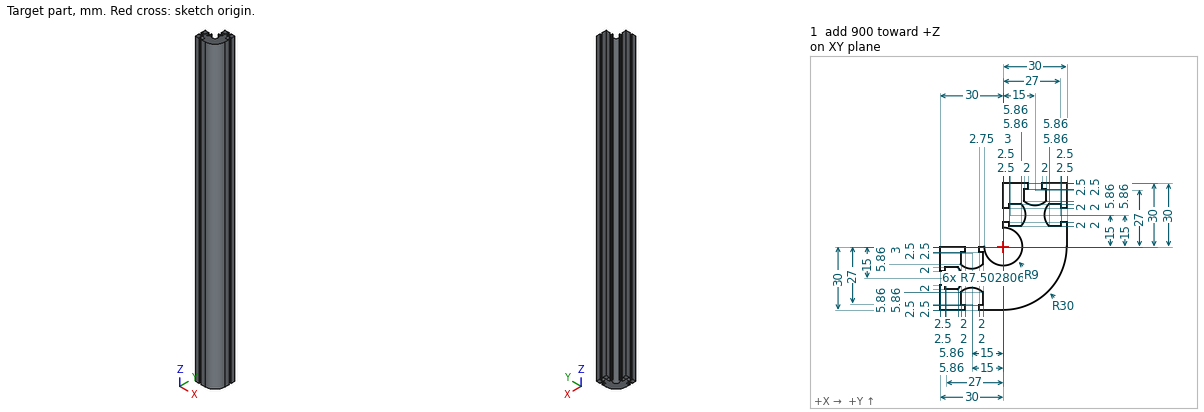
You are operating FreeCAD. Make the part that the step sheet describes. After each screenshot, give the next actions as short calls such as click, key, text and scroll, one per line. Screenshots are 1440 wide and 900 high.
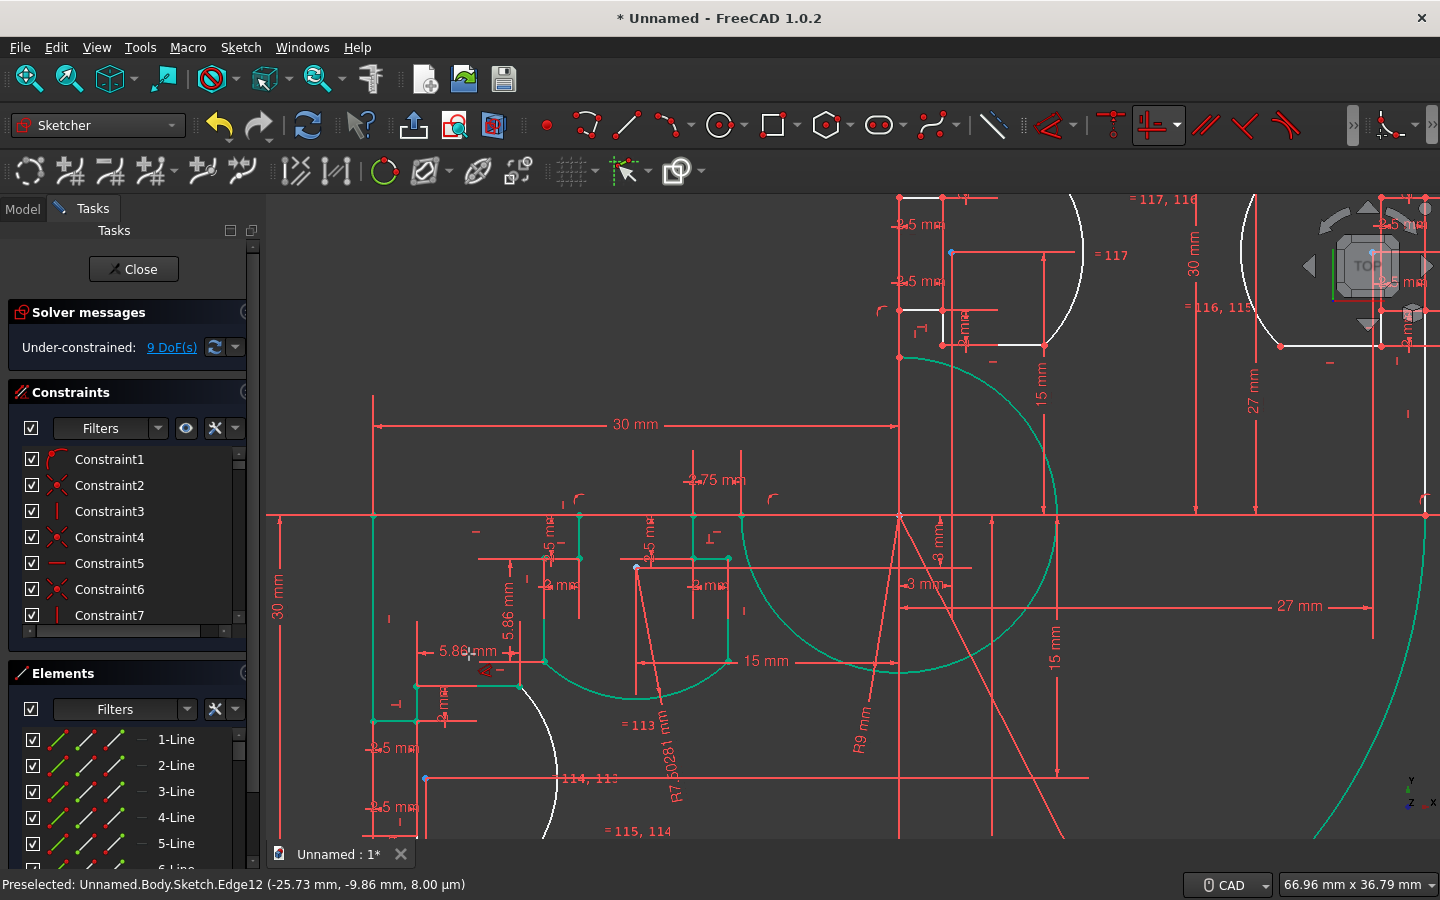
scroll(718, 517, down, 5)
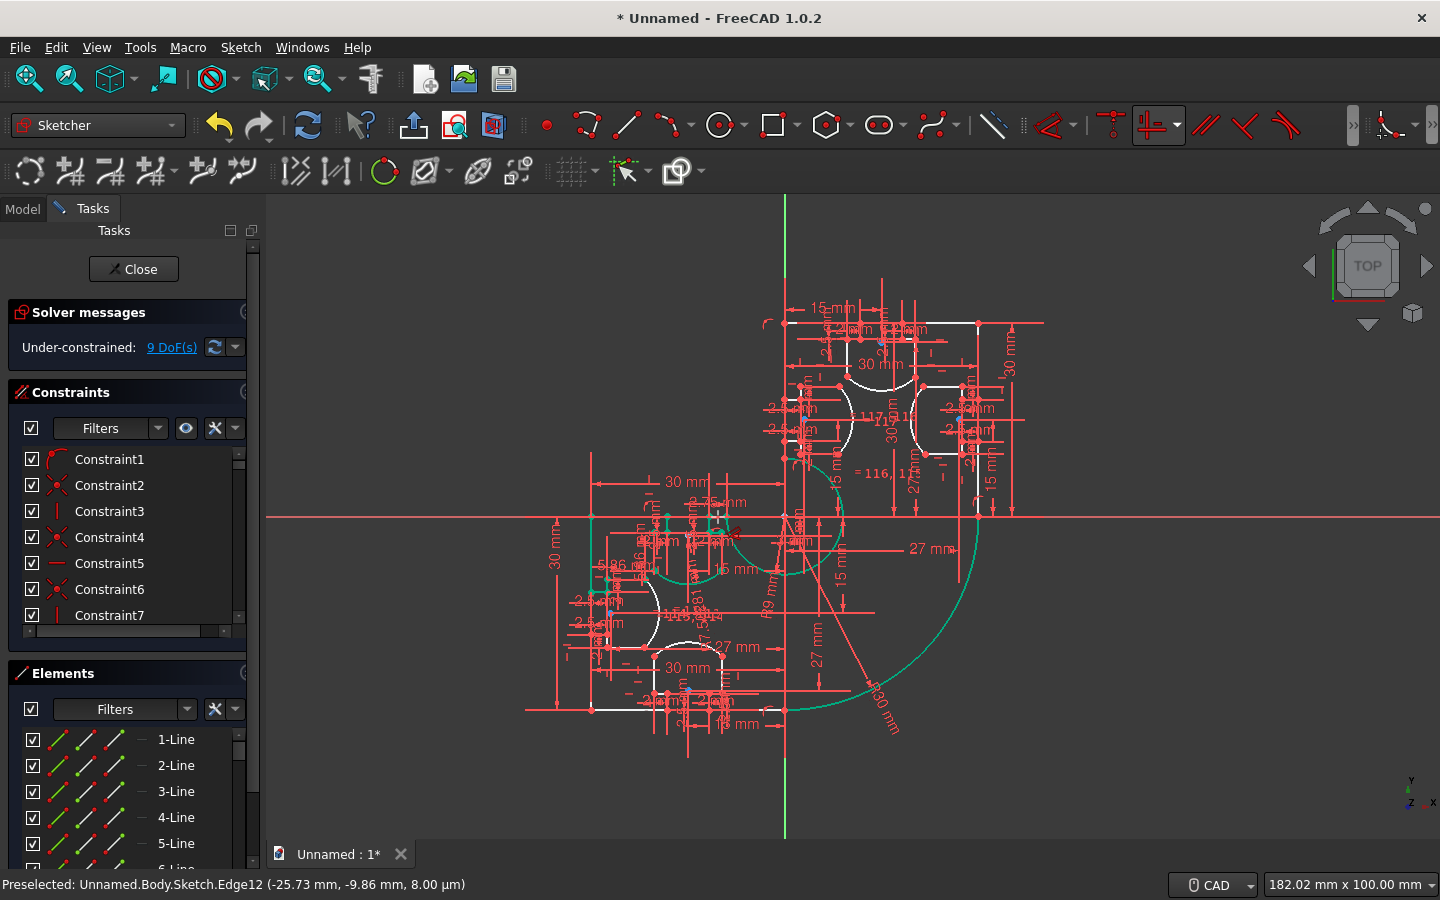
scroll(634, 648, up, 2)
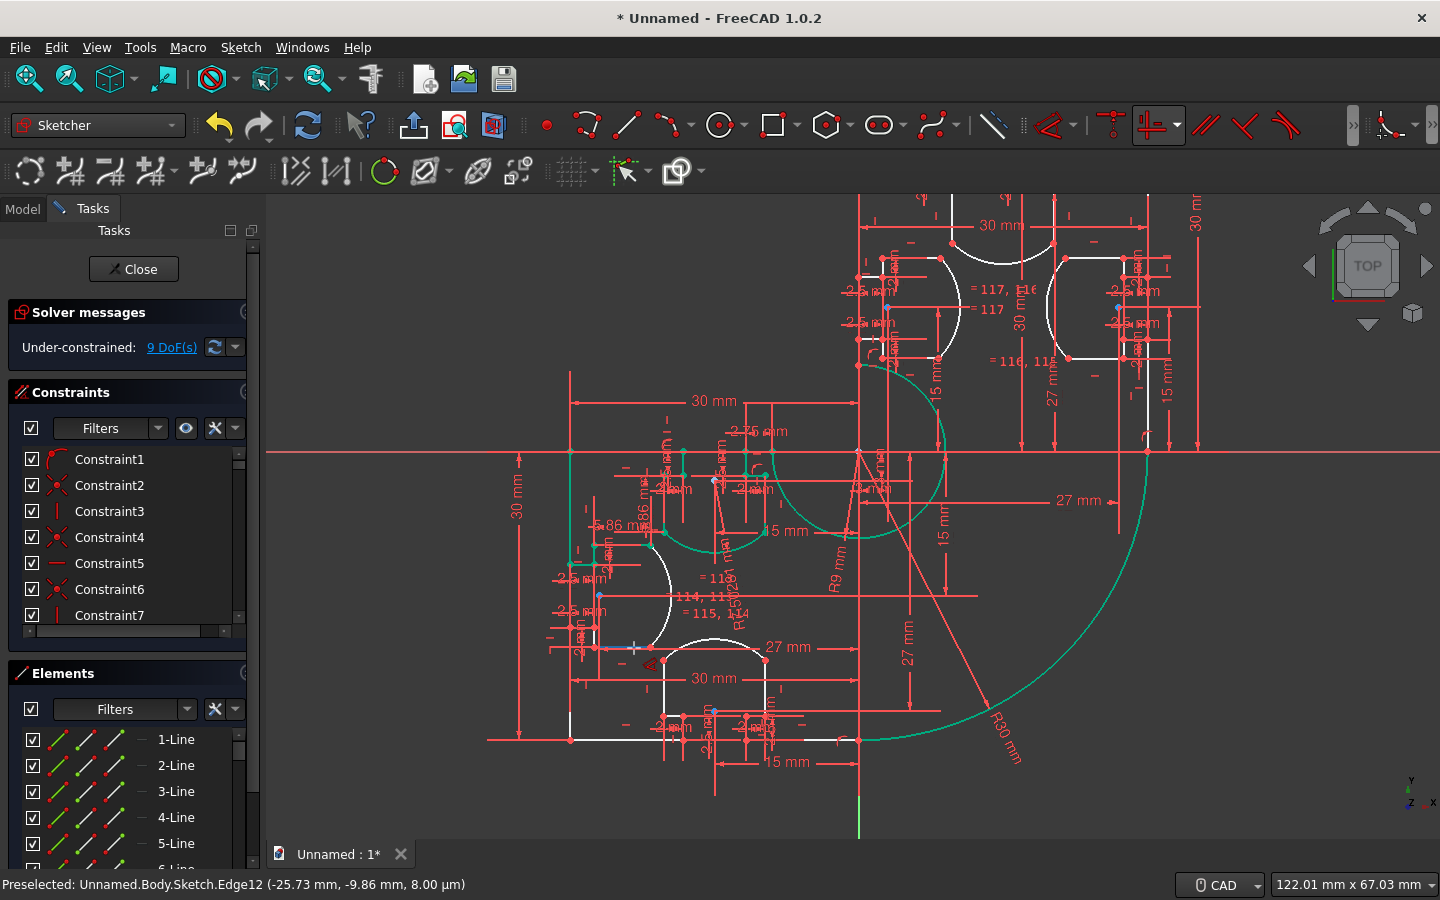
click(633, 647)
click(622, 681)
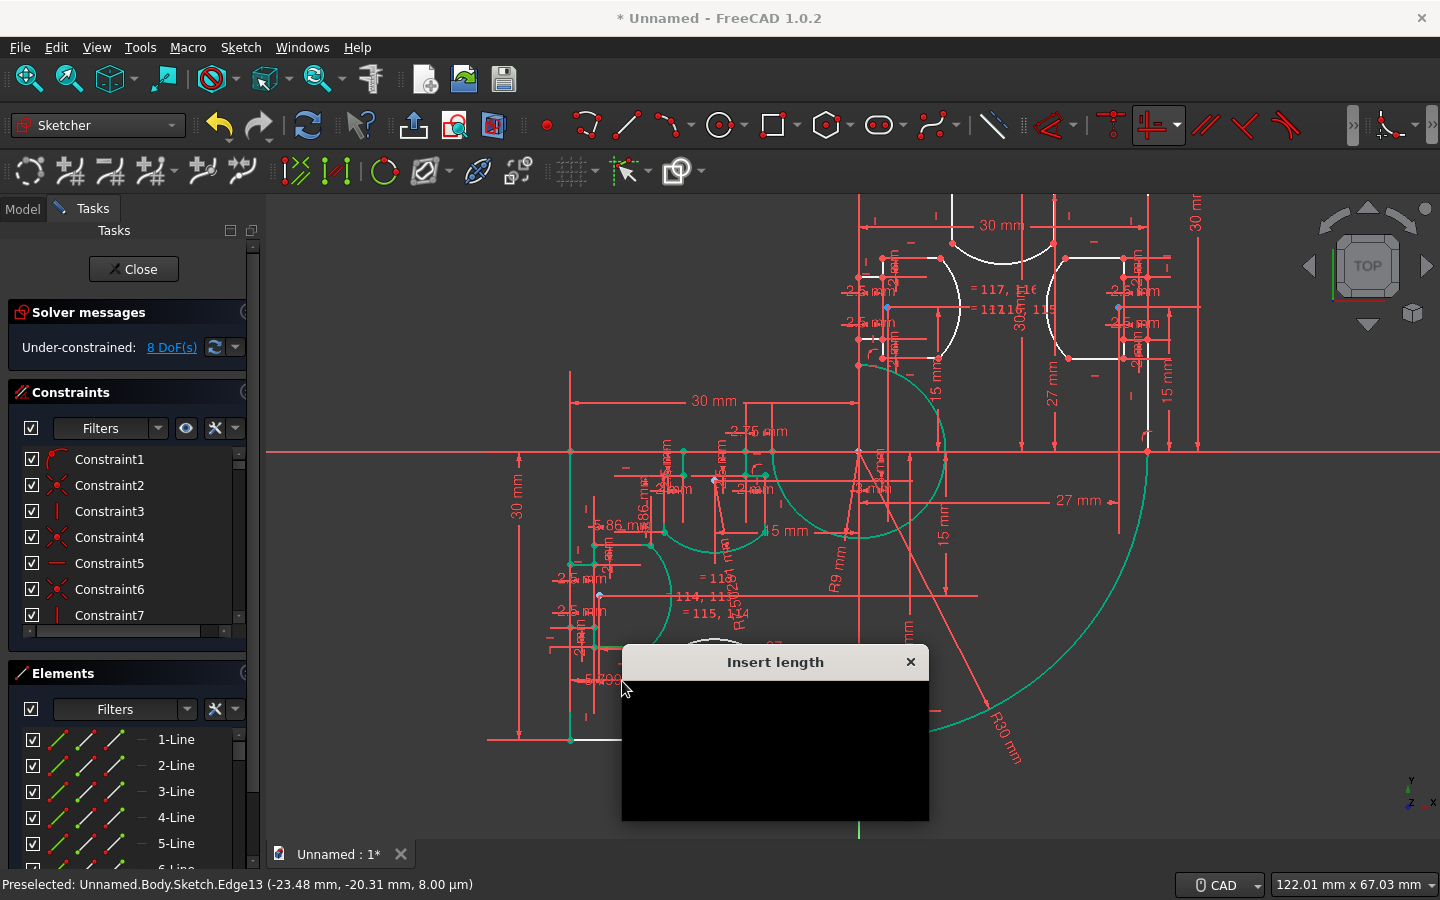
text(5.86)
key(Return)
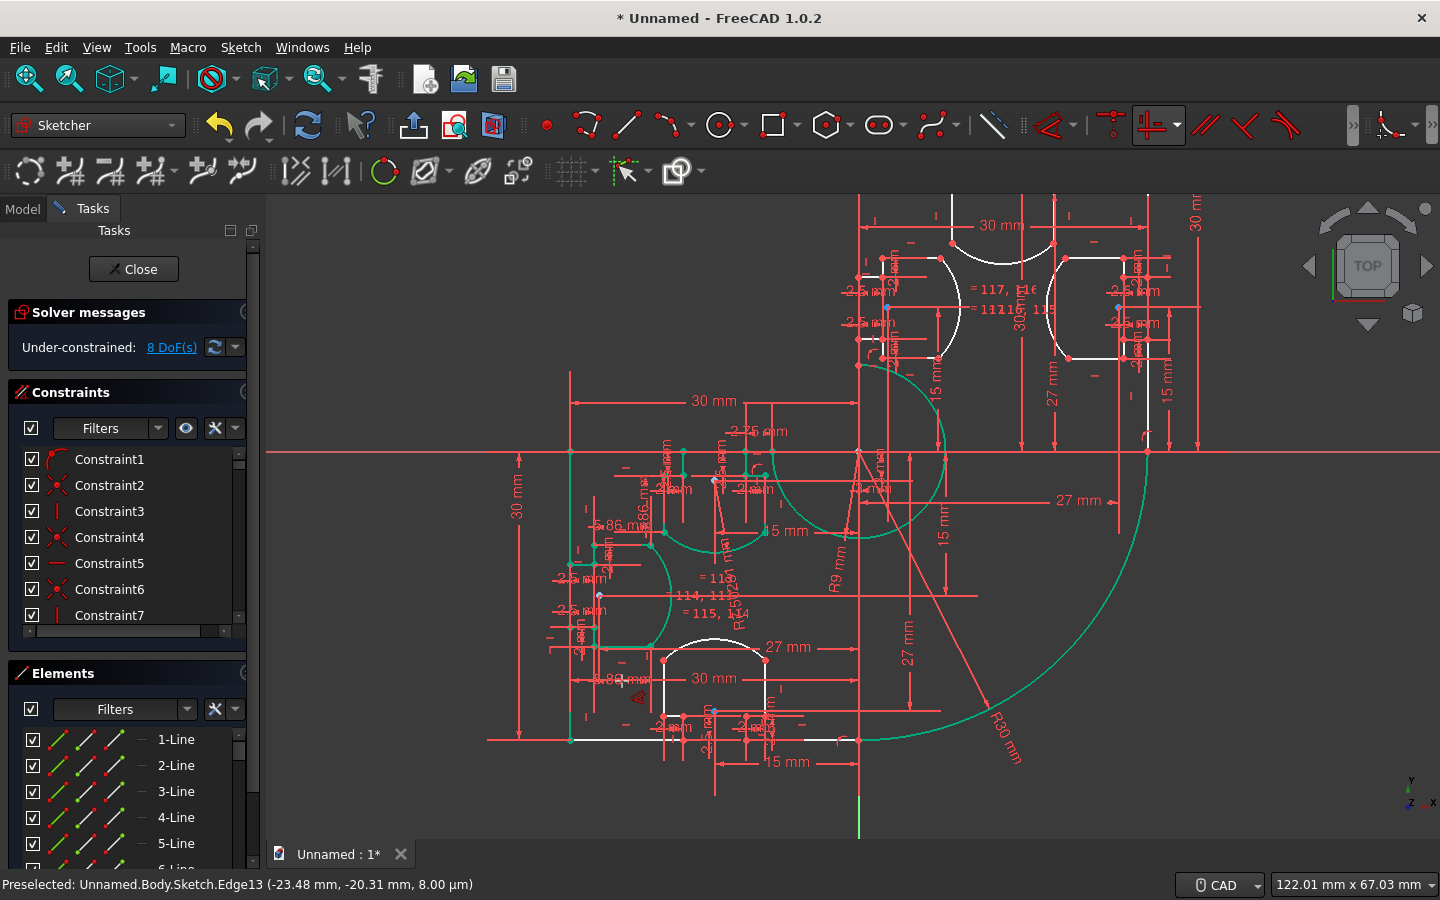
click(664, 699)
click(630, 708)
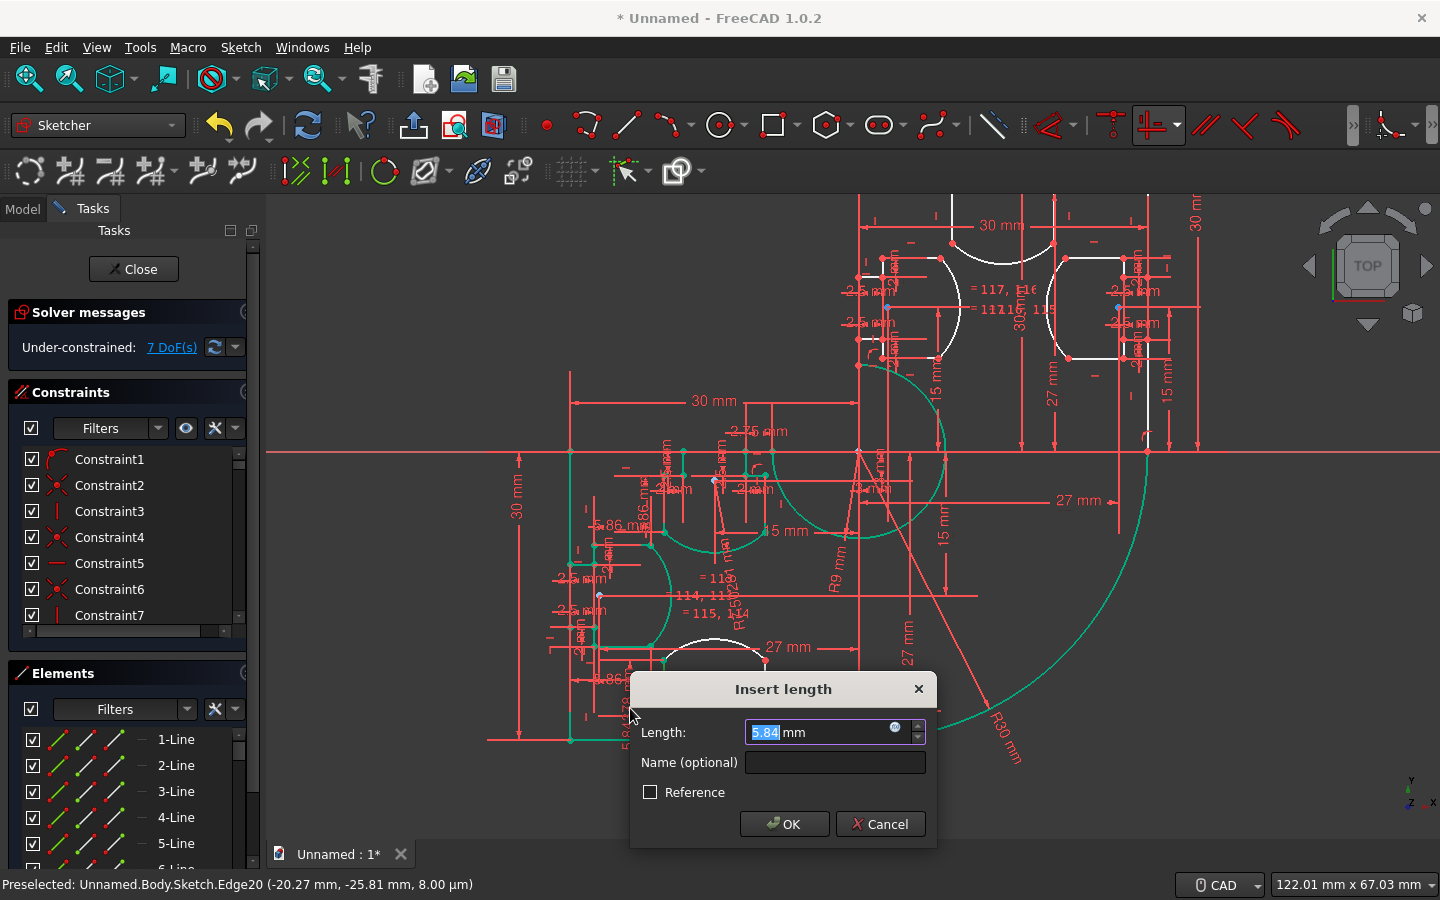
text(5.86)
key(Return)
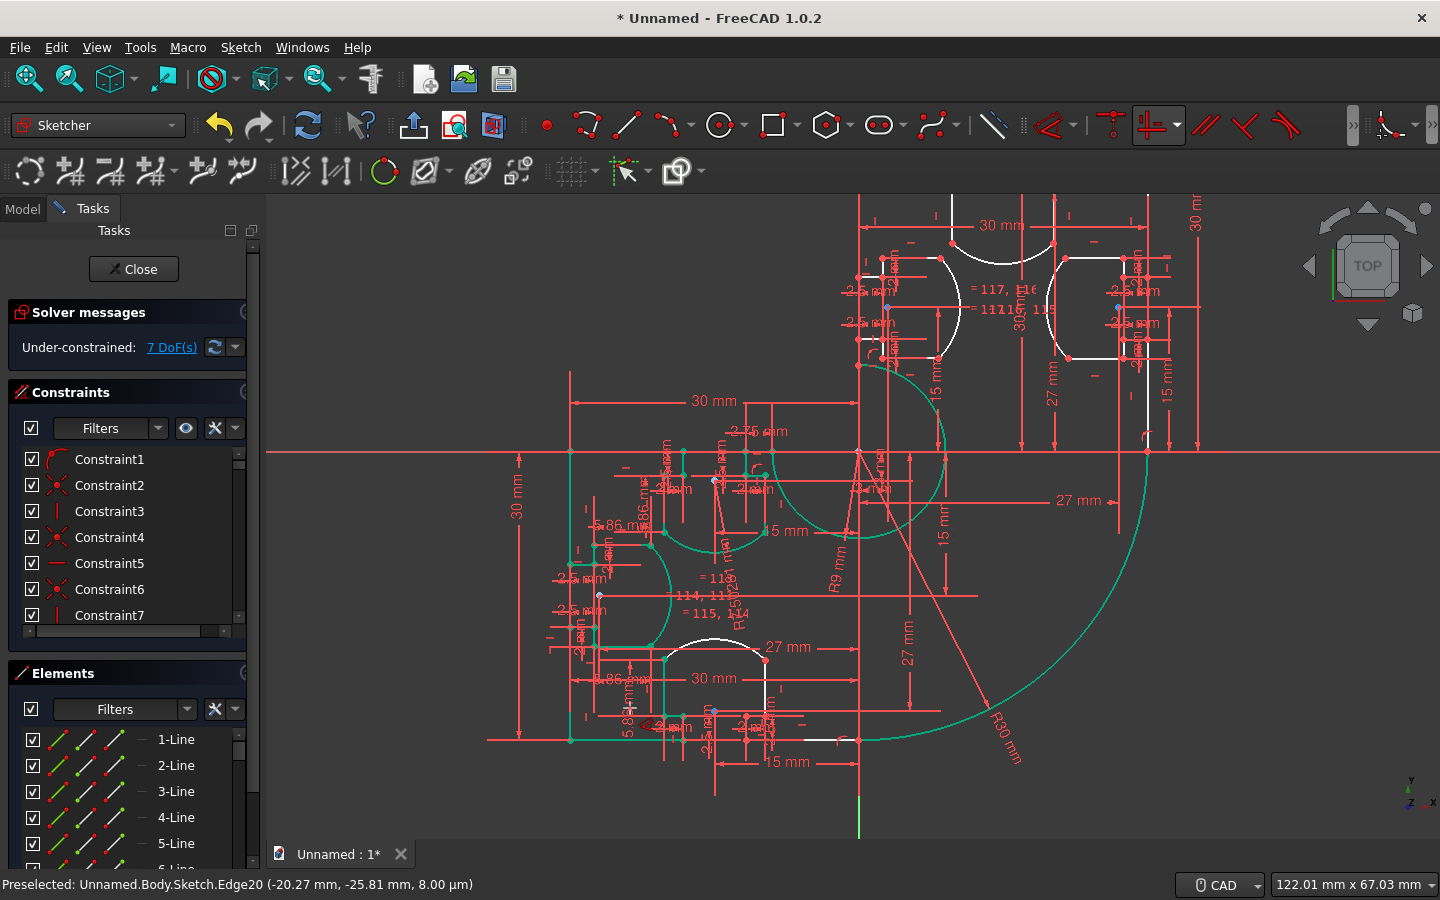
click(765, 677)
click(799, 688)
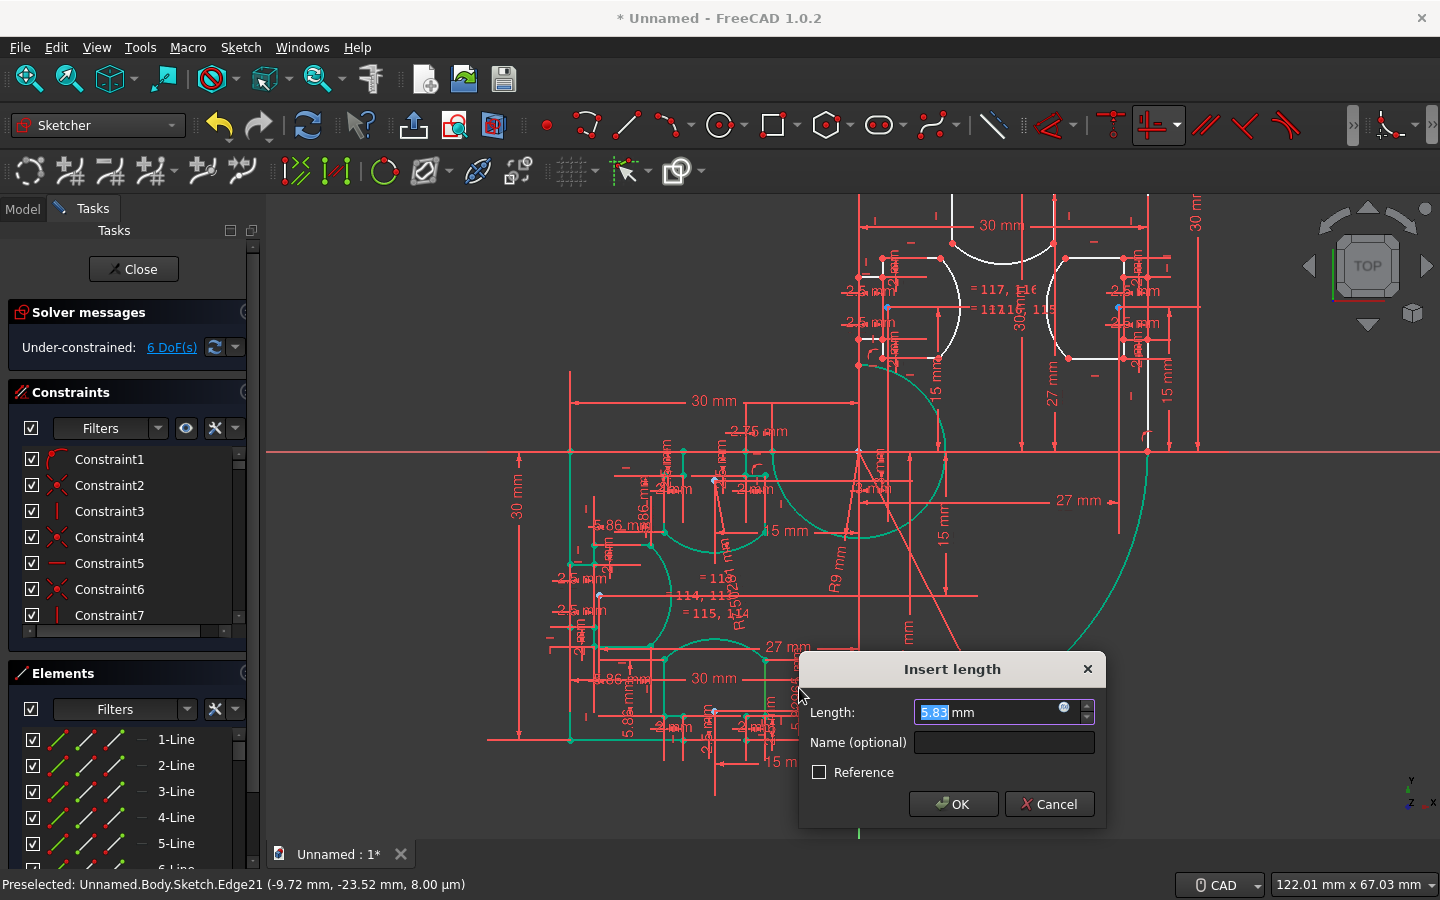
text(5.86)
key(Return)